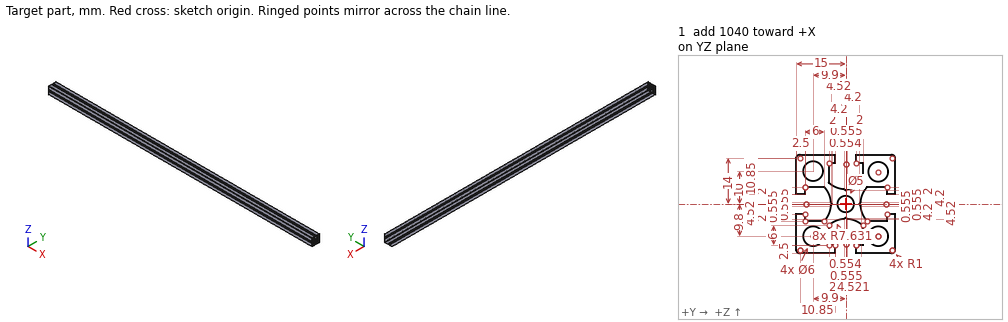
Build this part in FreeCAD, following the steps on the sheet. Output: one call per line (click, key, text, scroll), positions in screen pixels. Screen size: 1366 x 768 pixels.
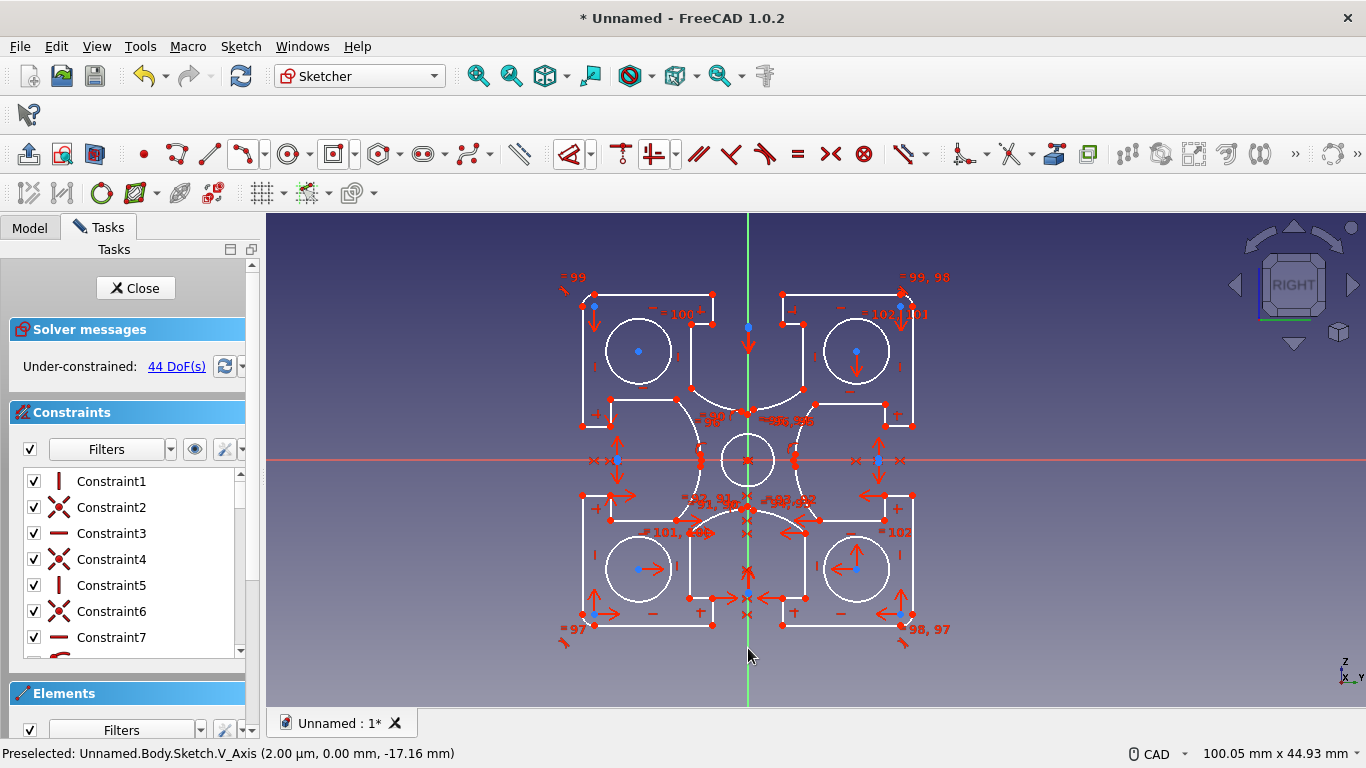
click(611, 400)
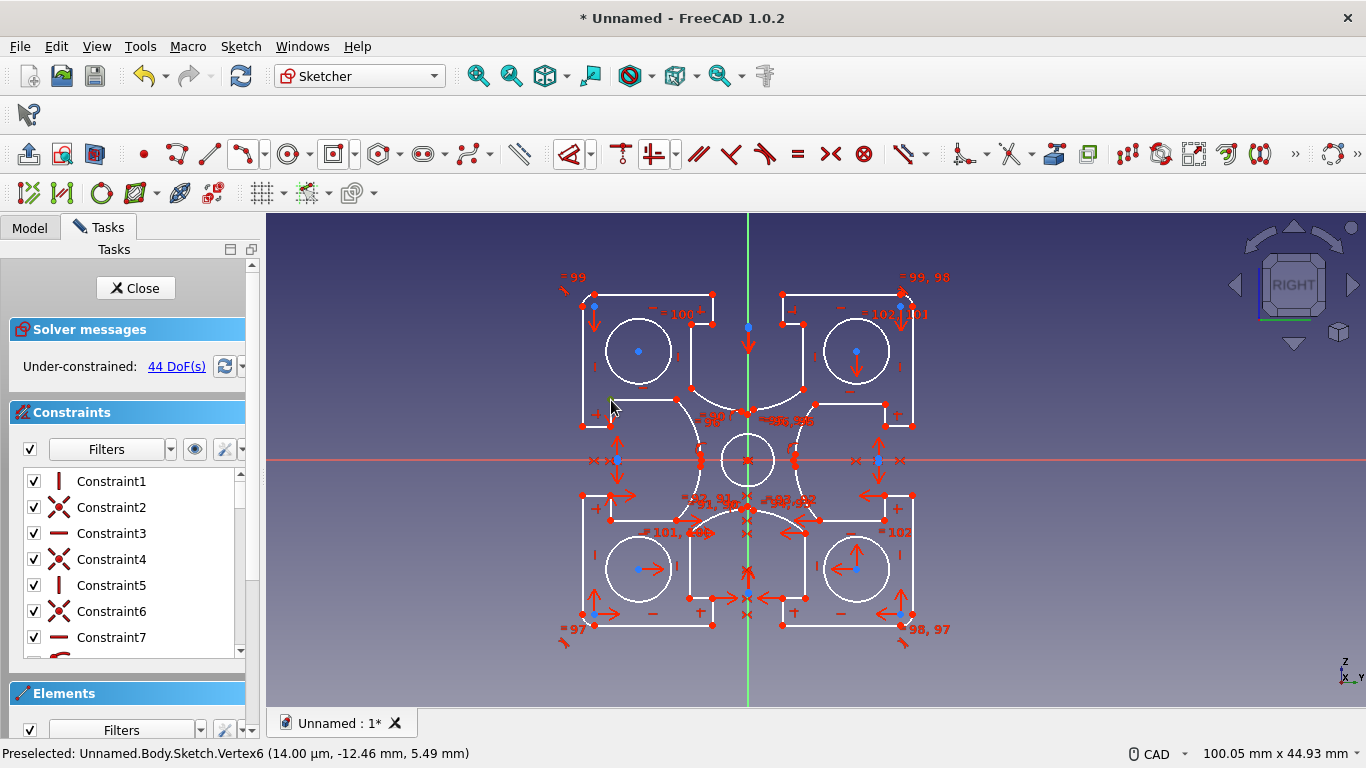
click(885, 404)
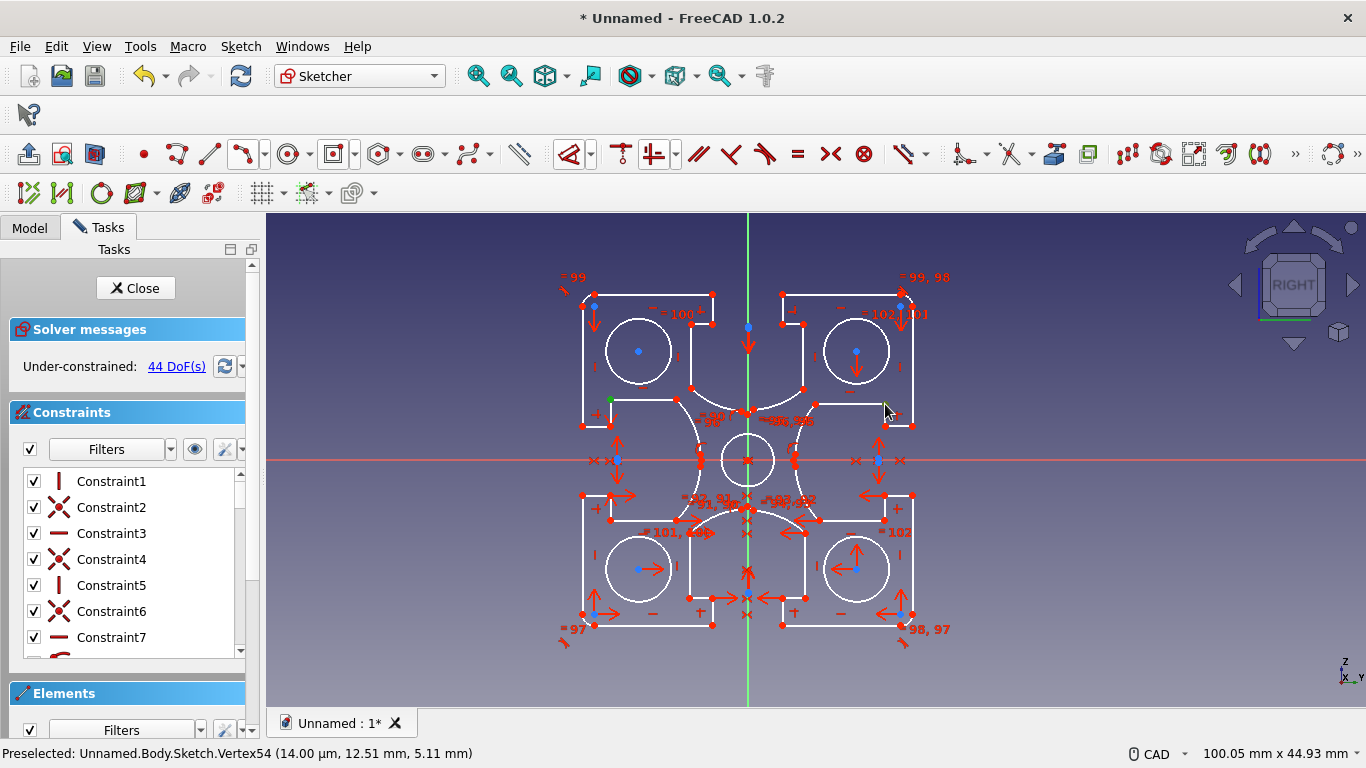
click(748, 648)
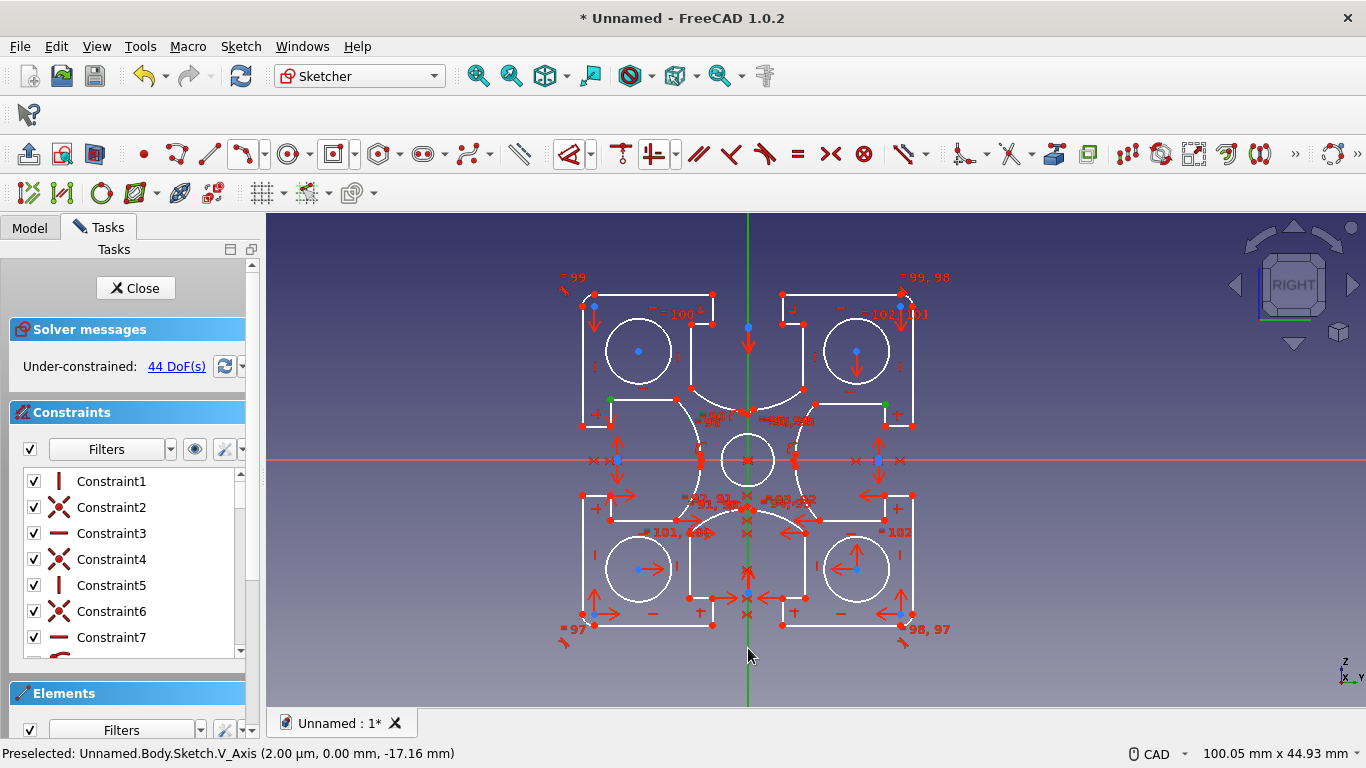
click(831, 154)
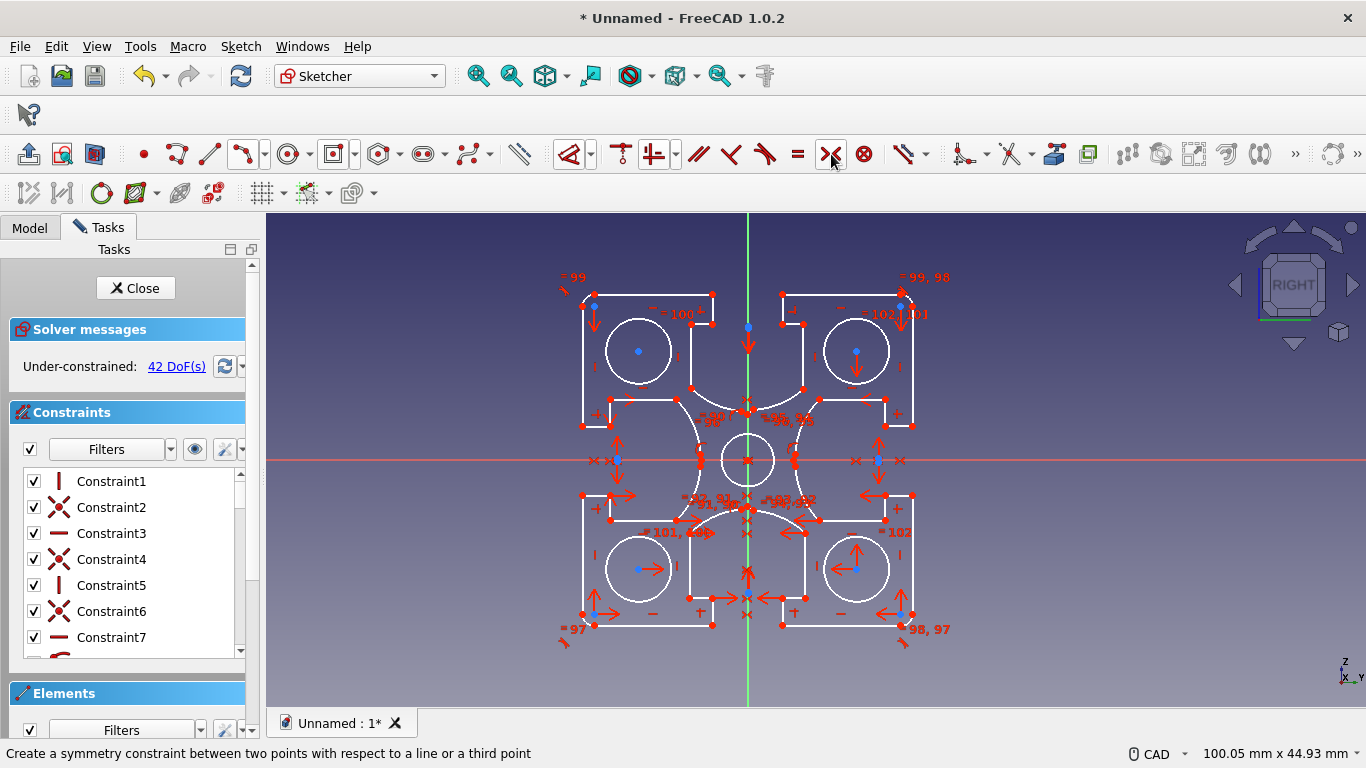
click(783, 598)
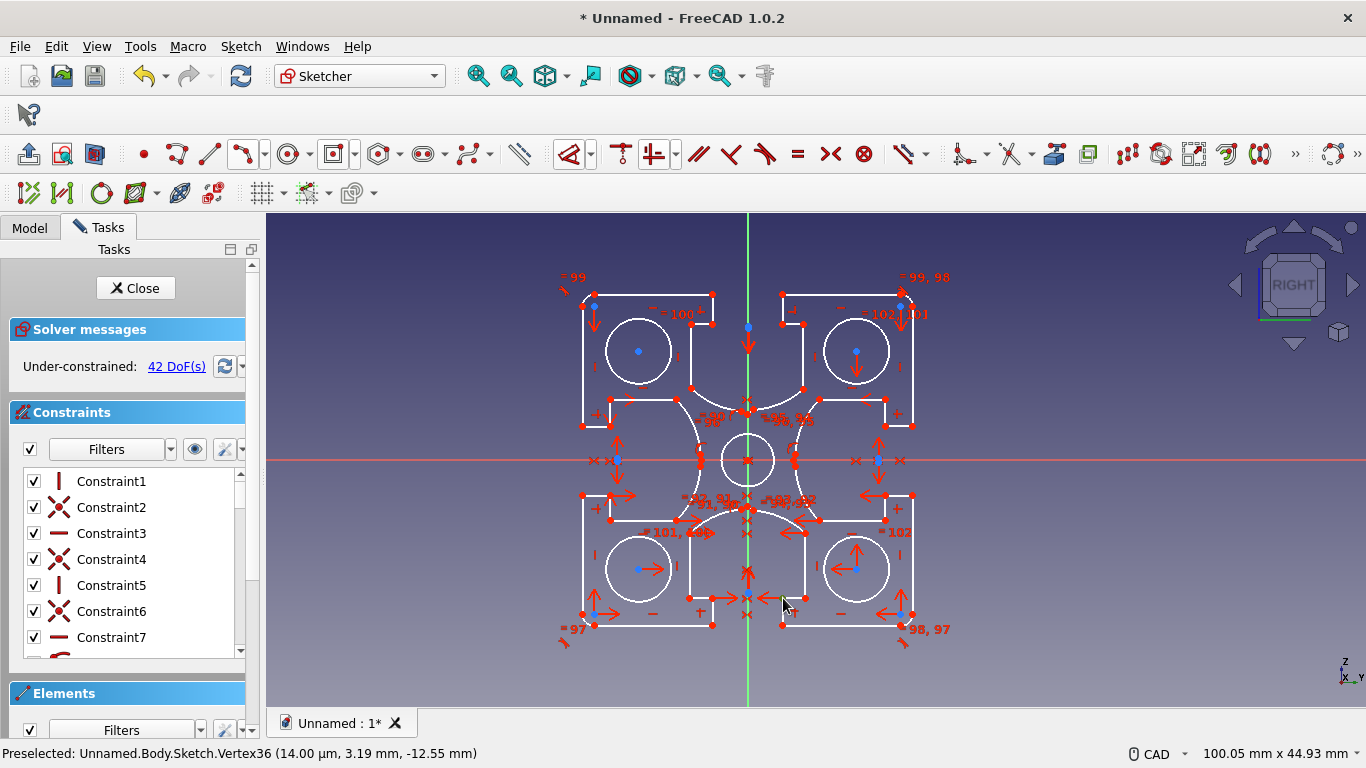
click(783, 324)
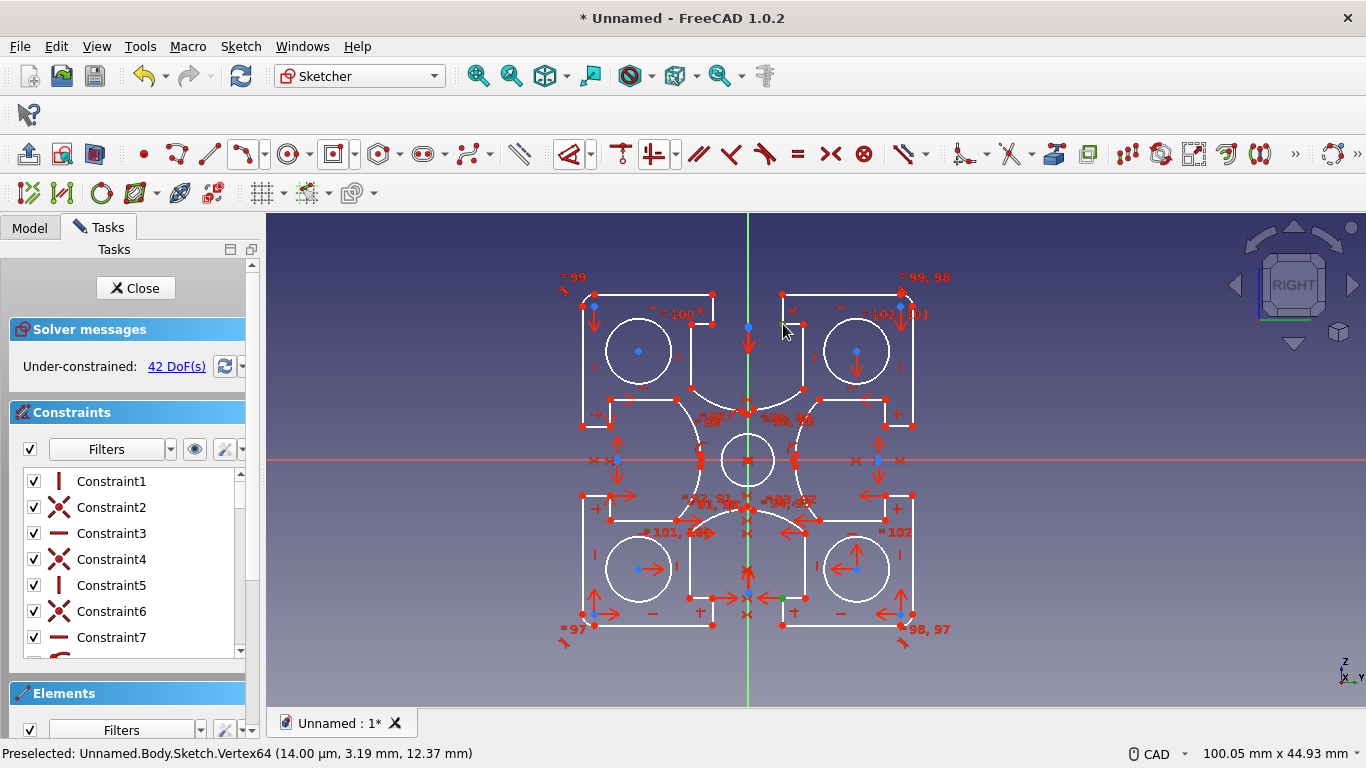
click(359, 460)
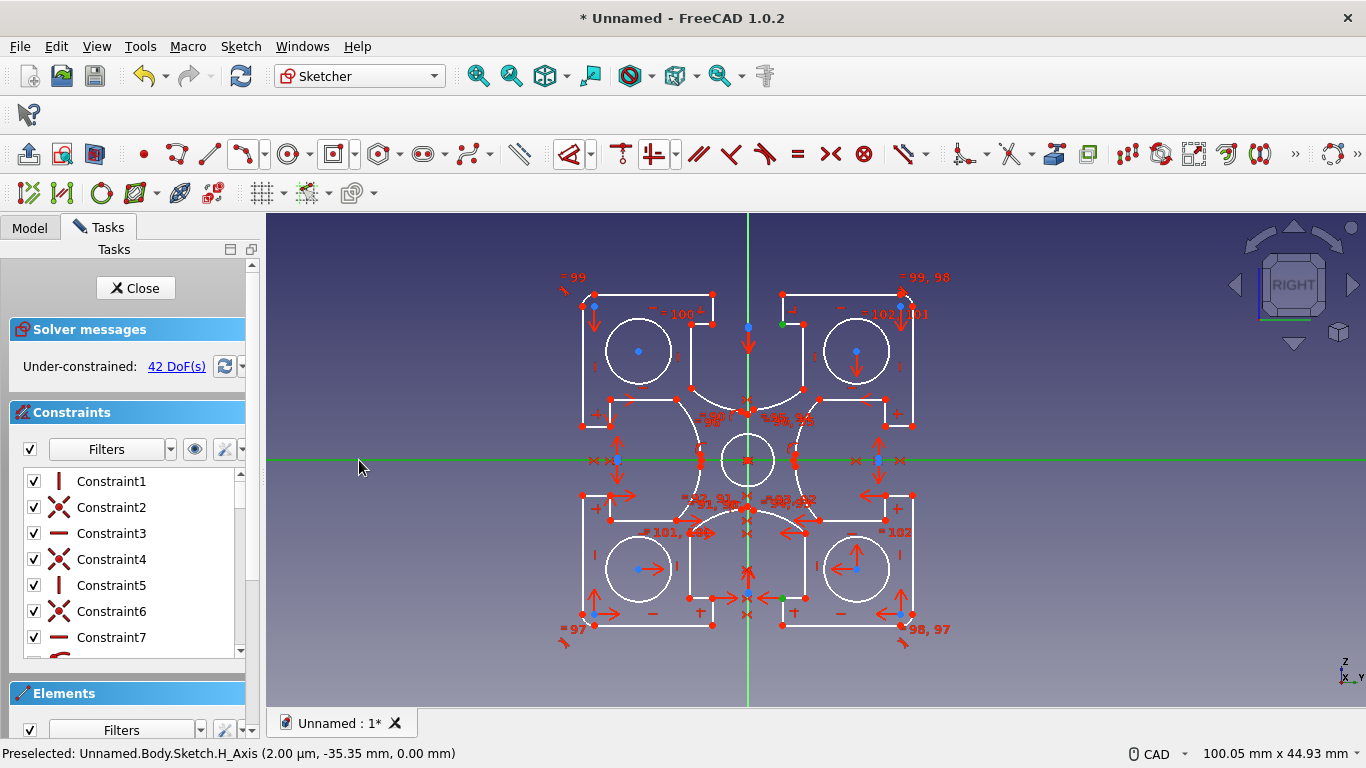
key(s)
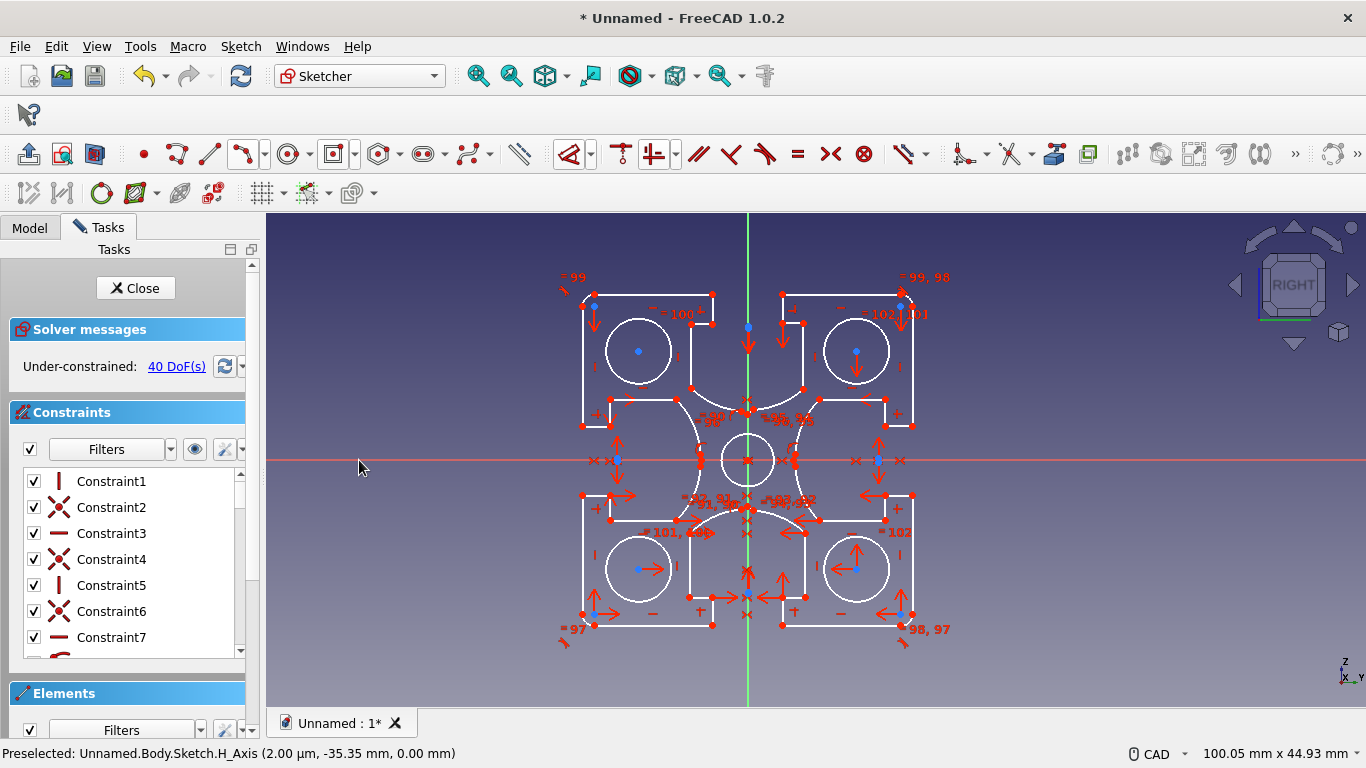
click(690, 598)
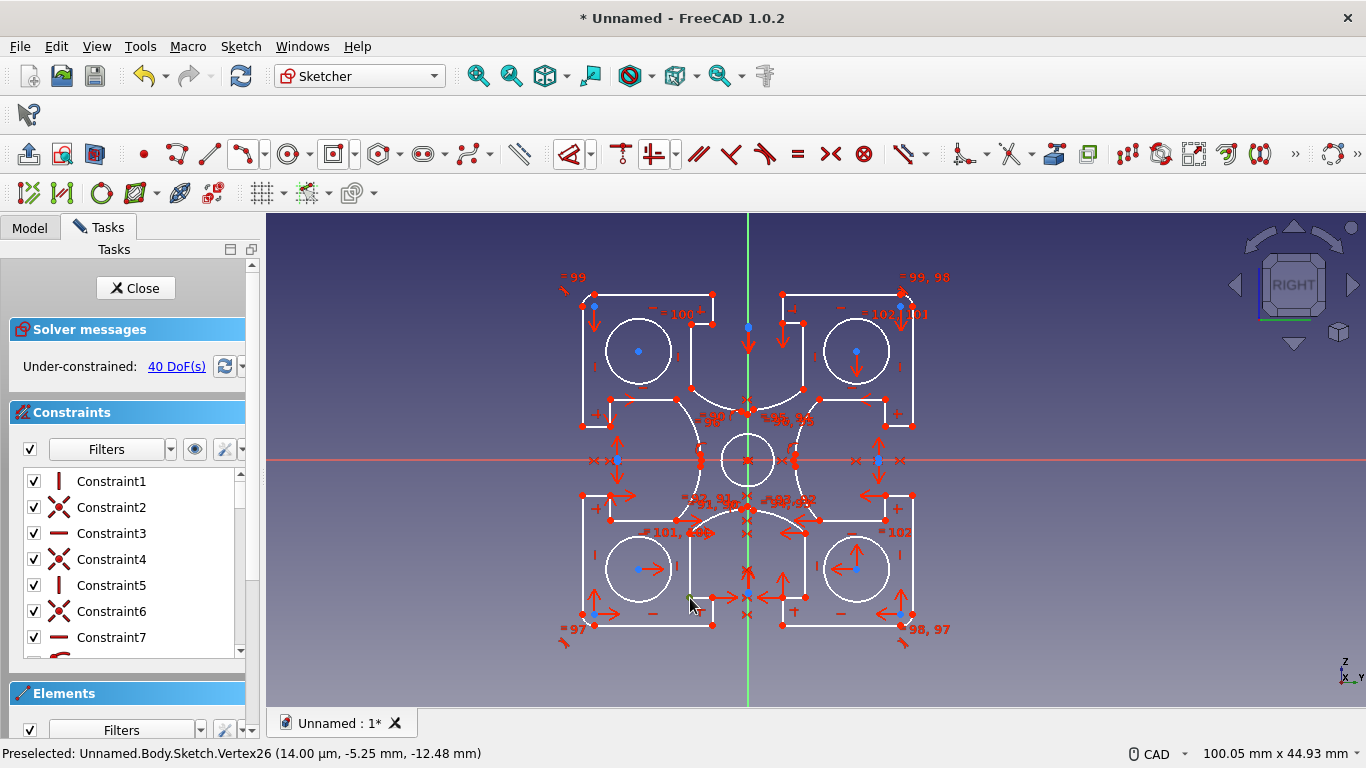
click(691, 324)